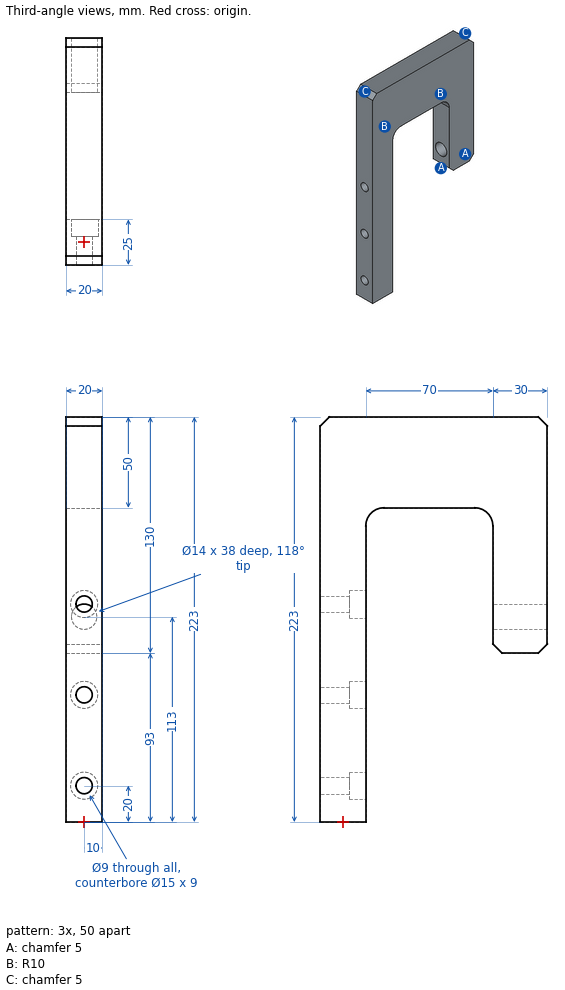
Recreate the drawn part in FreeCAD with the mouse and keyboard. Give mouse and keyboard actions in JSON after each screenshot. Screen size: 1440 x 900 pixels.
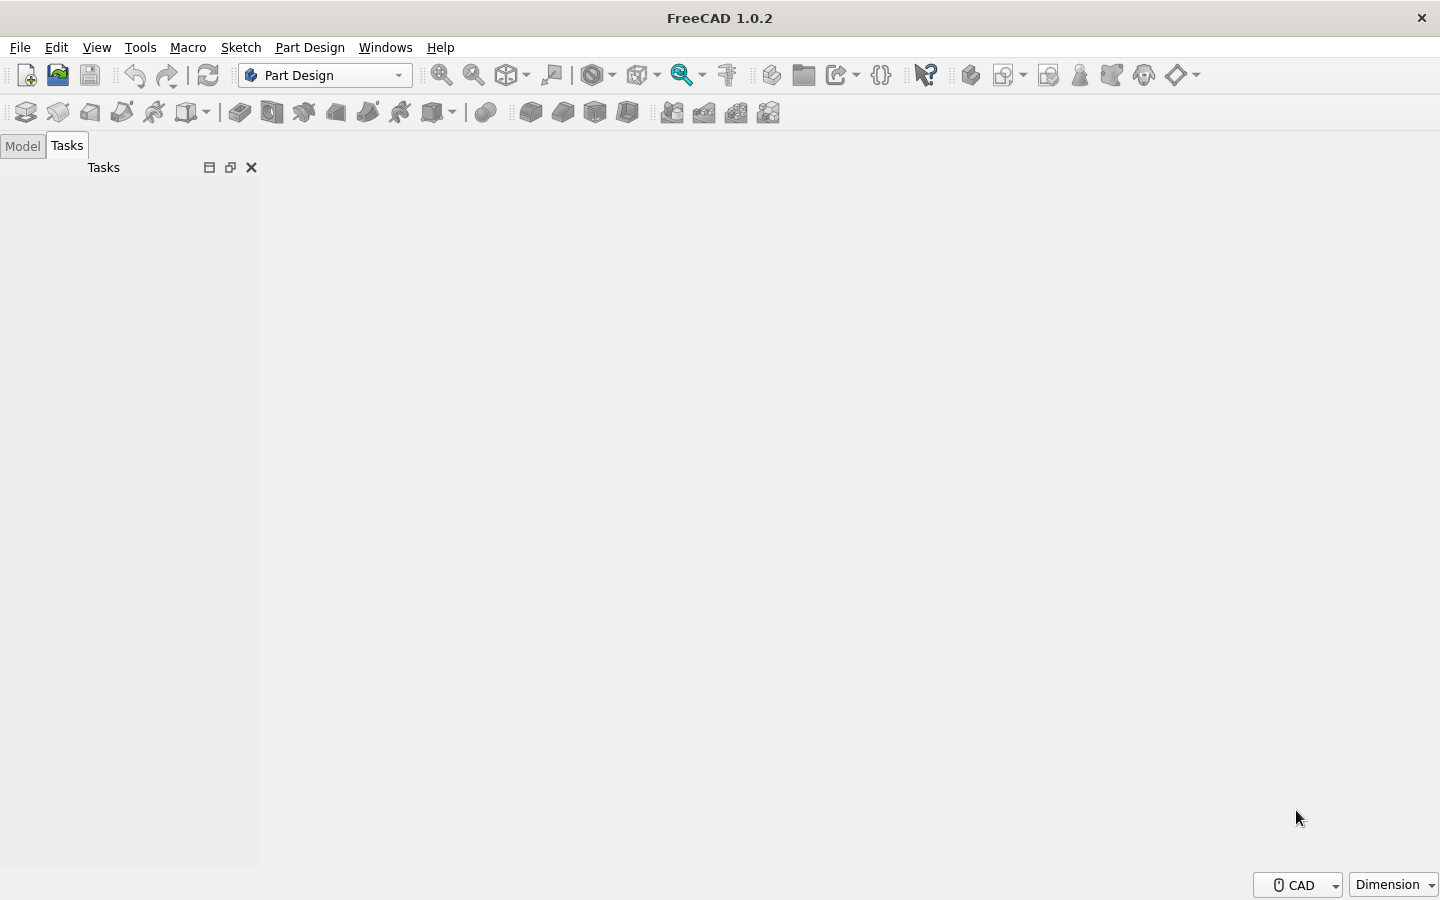
{"action": "left_click", "coordinate": [26, 76]}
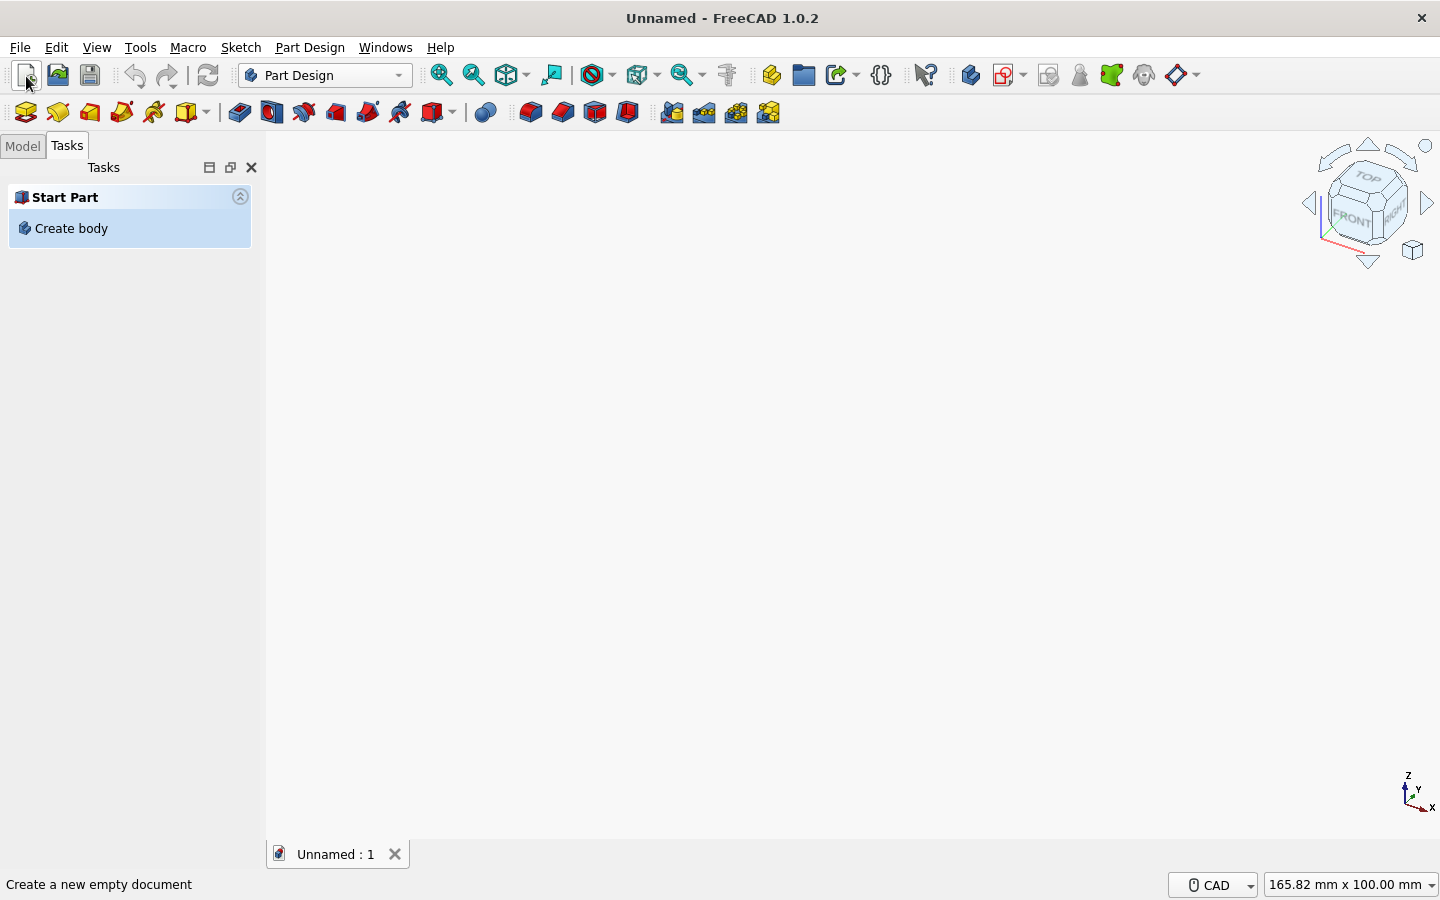
{"action": "left_click", "coordinate": [1004, 76]}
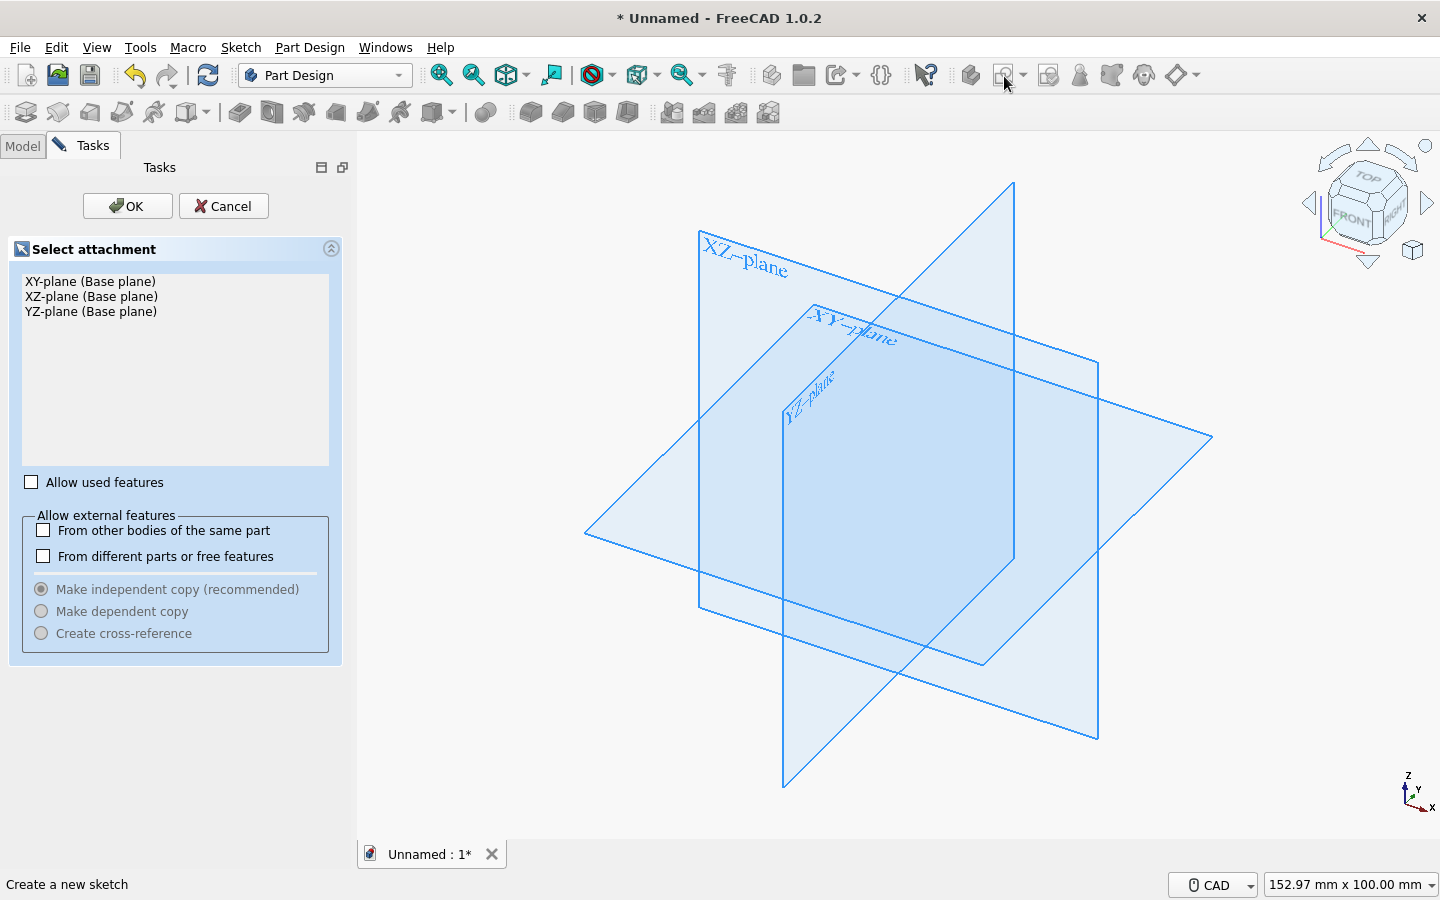
{"action": "left_click", "coordinate": [82, 282]}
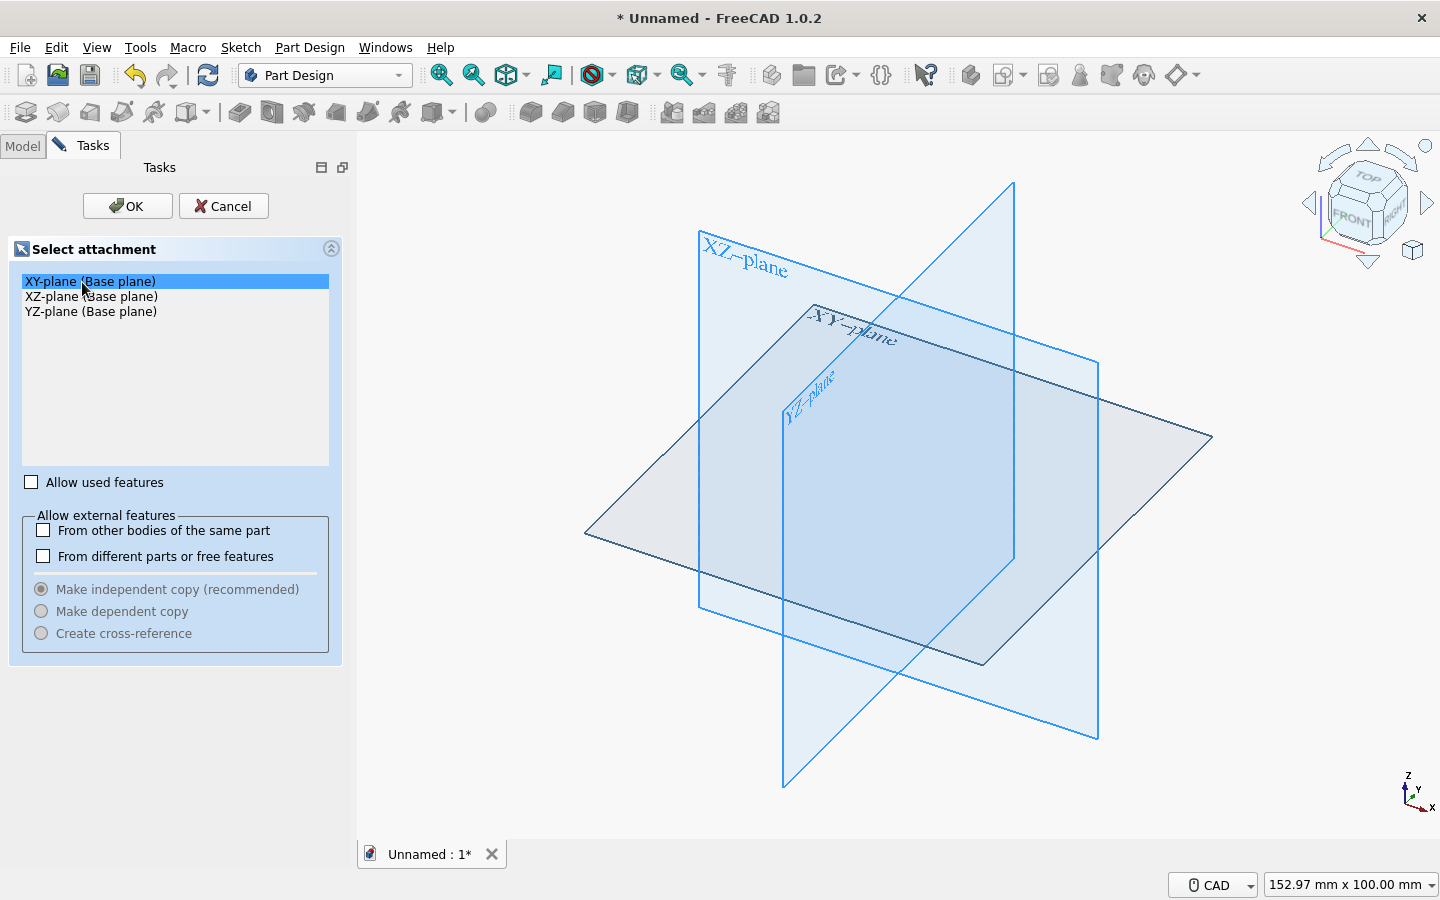
{"action": "left_click", "coordinate": [128, 206]}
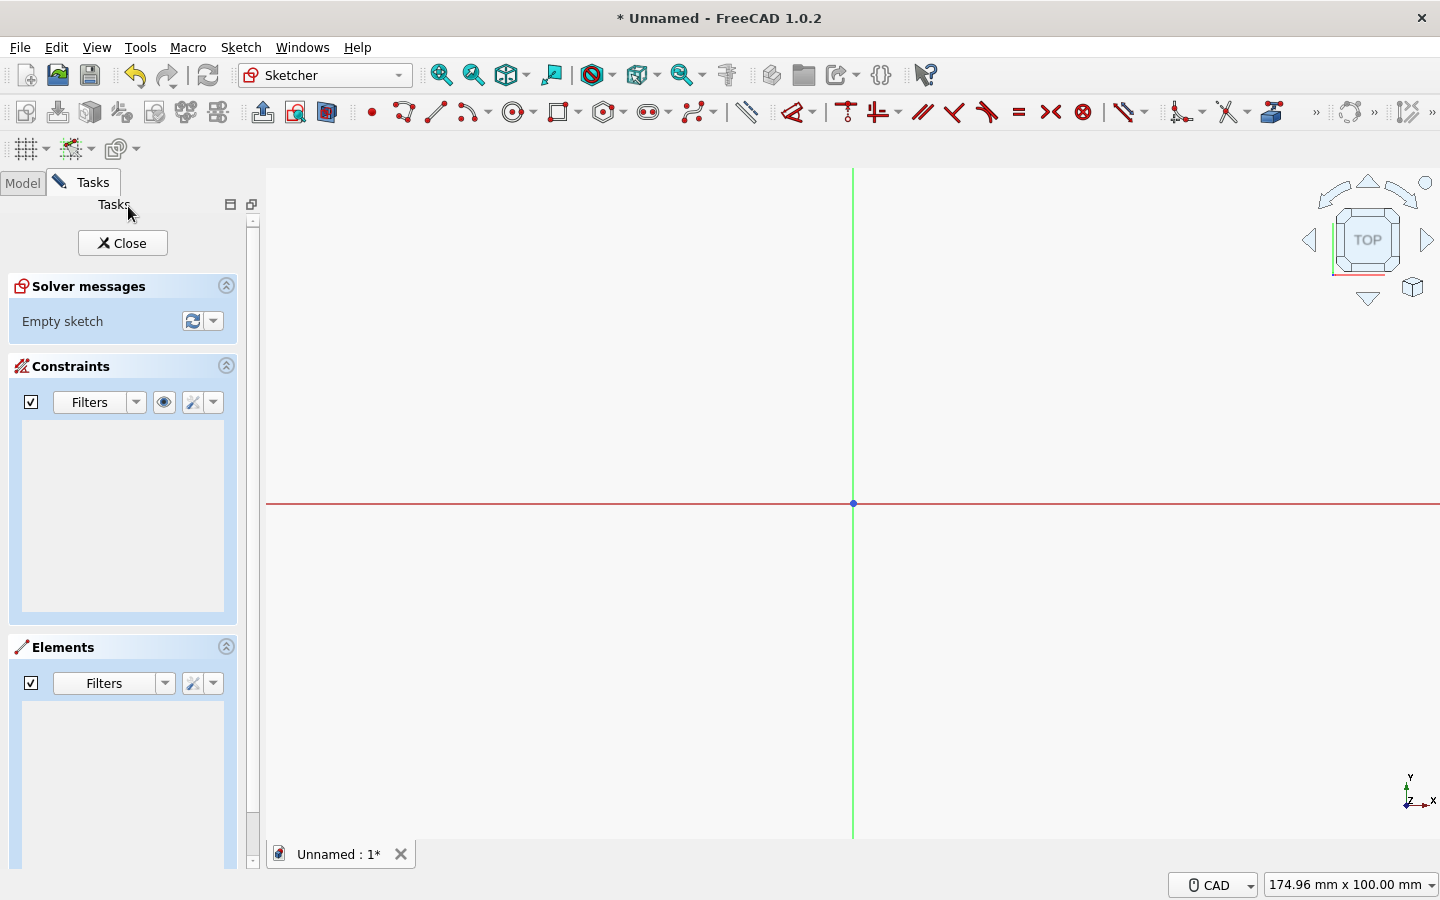
{"action": "scroll", "coordinate": [893, 504], "scroll_direction": "up", "scroll_amount": 5}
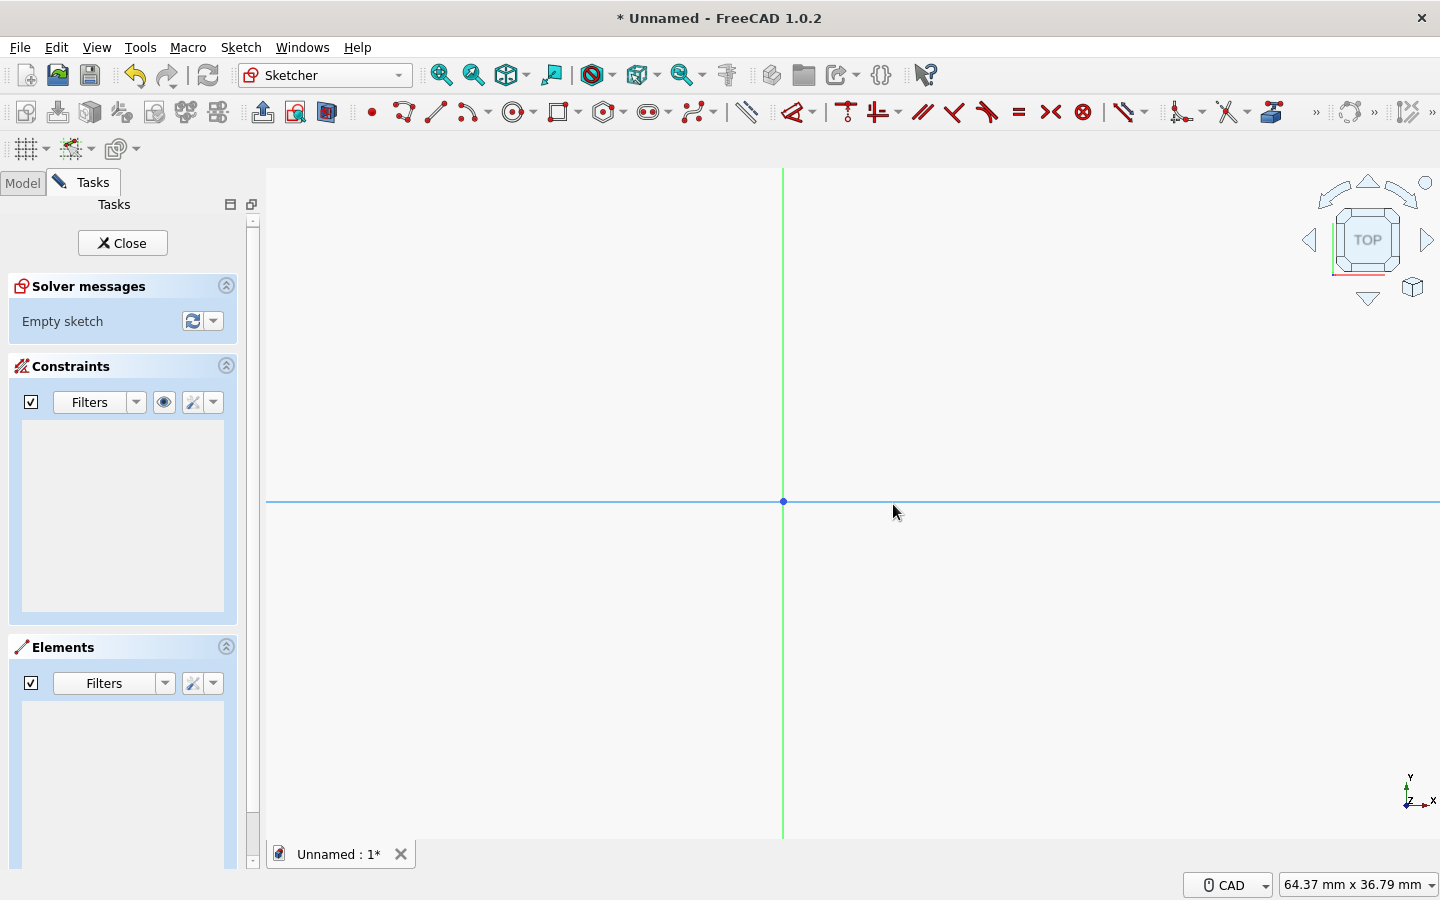
{"action": "key", "text": "g v"}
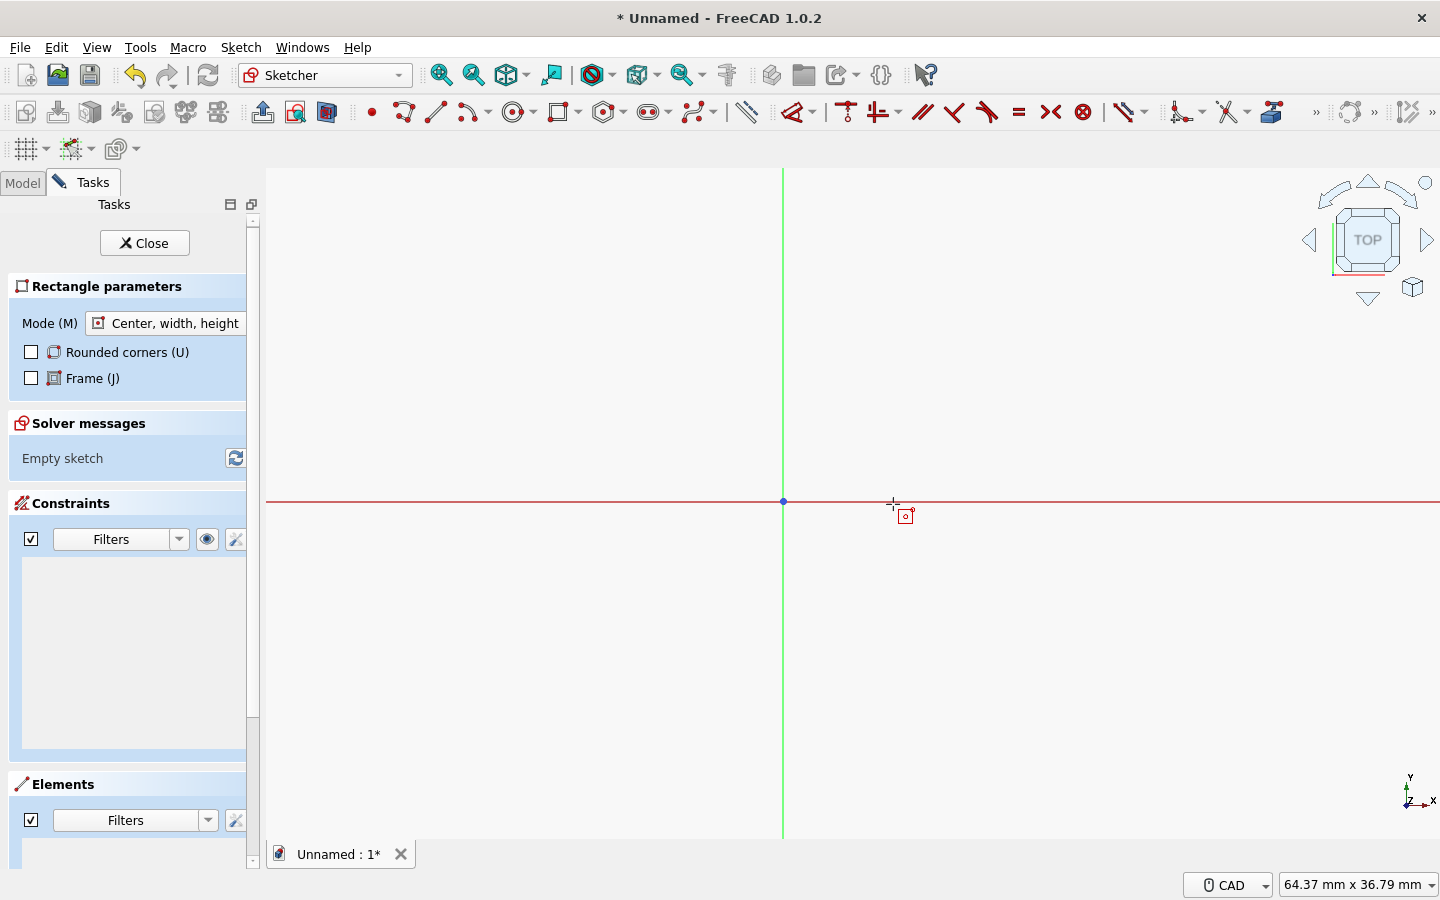
{"action": "left_click", "coordinate": [783, 502]}
{"action": "left_click", "coordinate": [966, 274]}
{"action": "key", "text": "Escape"}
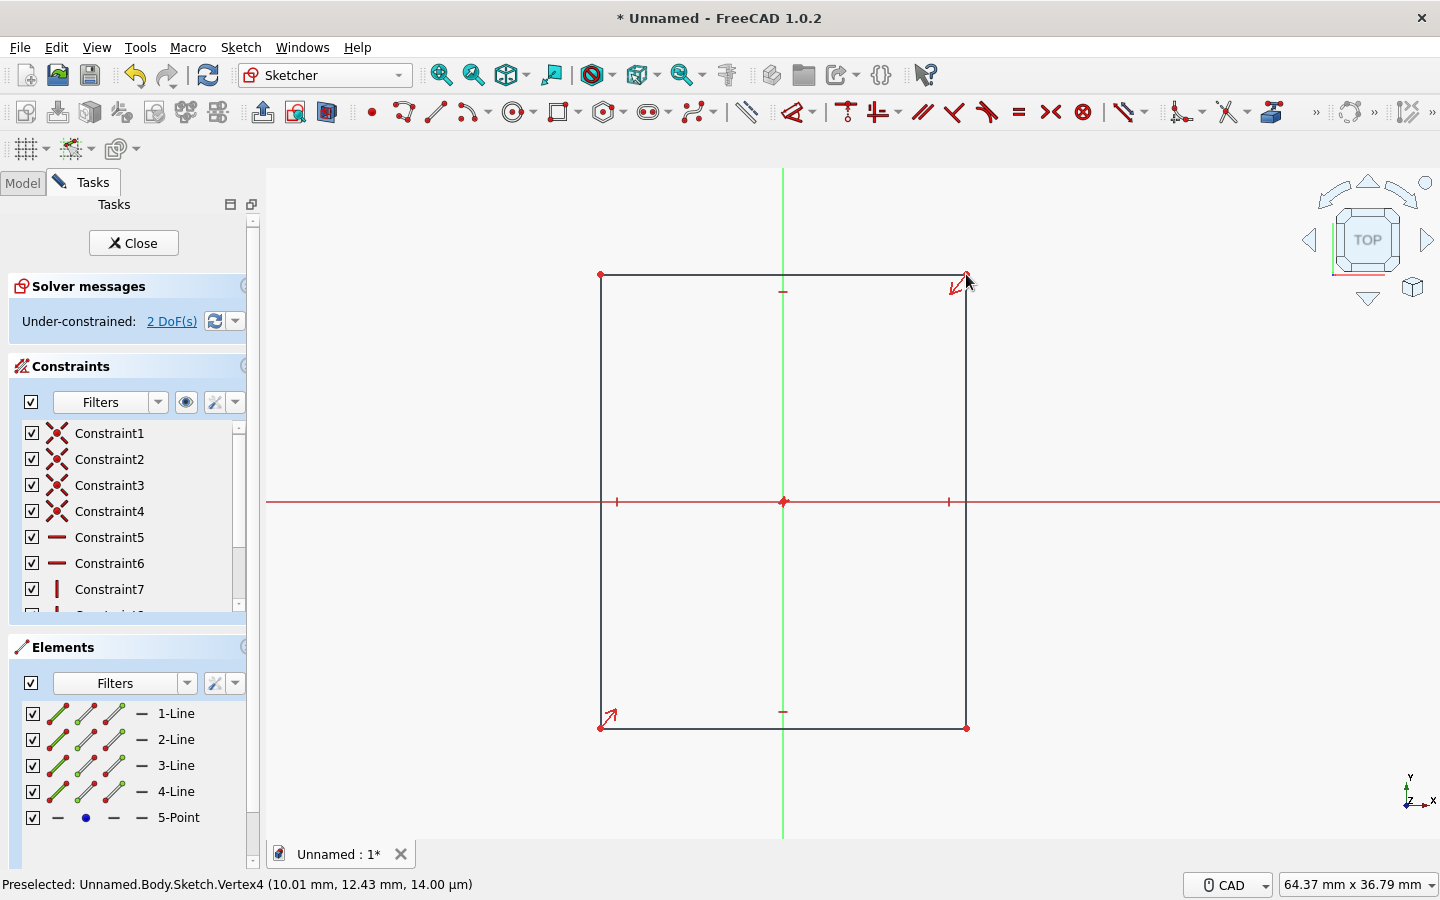
{"action": "left_click", "coordinate": [792, 112]}